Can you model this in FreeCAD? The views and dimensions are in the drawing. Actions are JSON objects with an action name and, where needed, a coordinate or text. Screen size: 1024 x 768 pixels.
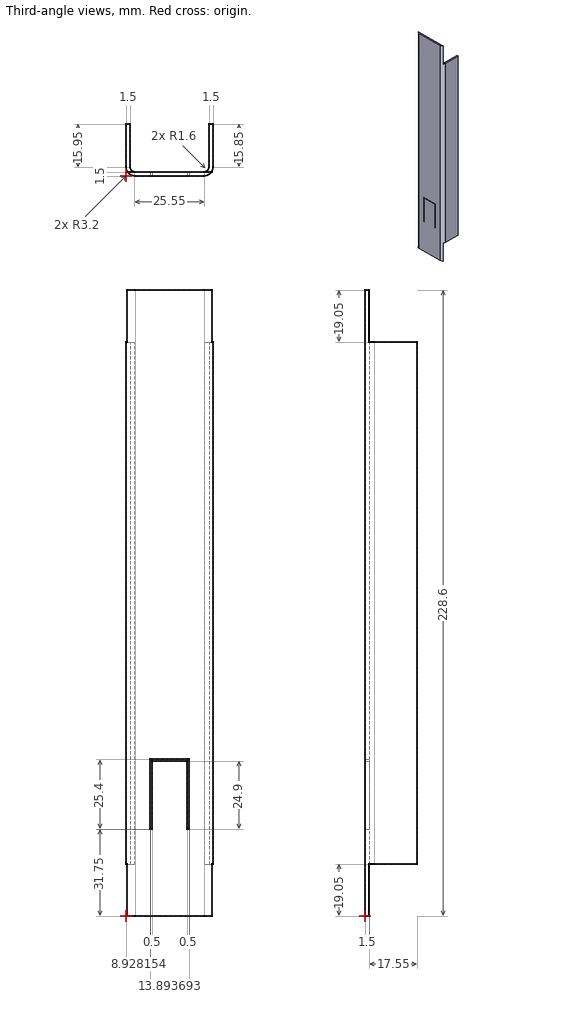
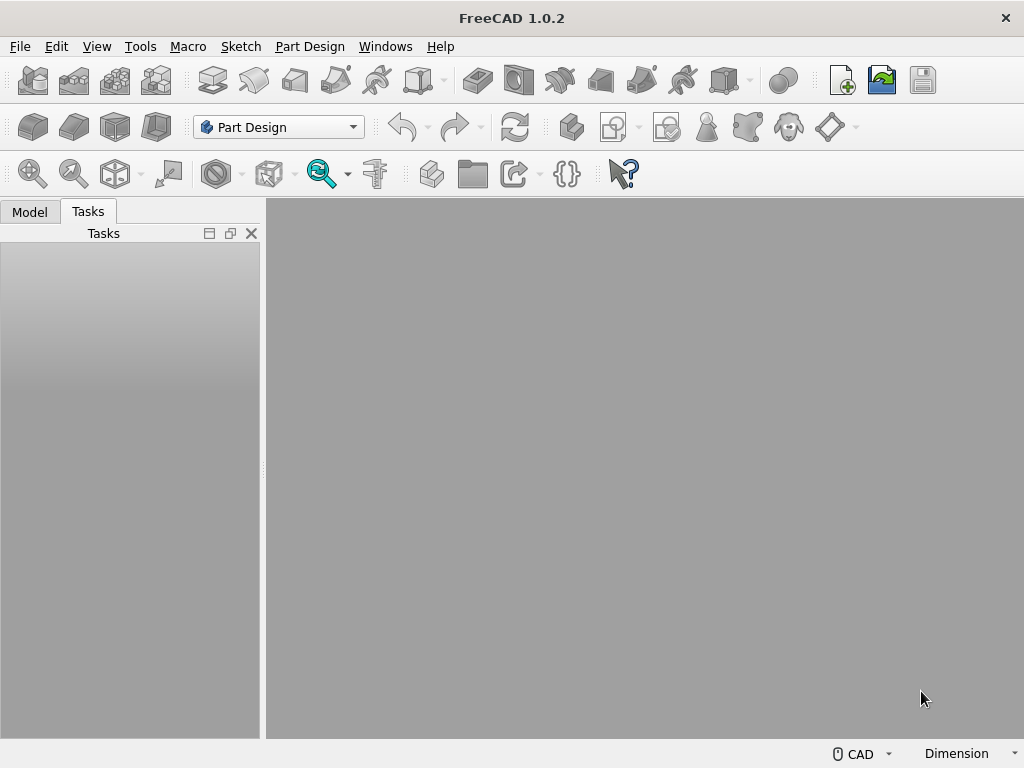
{"action": "left_click", "coordinate": [841, 80]}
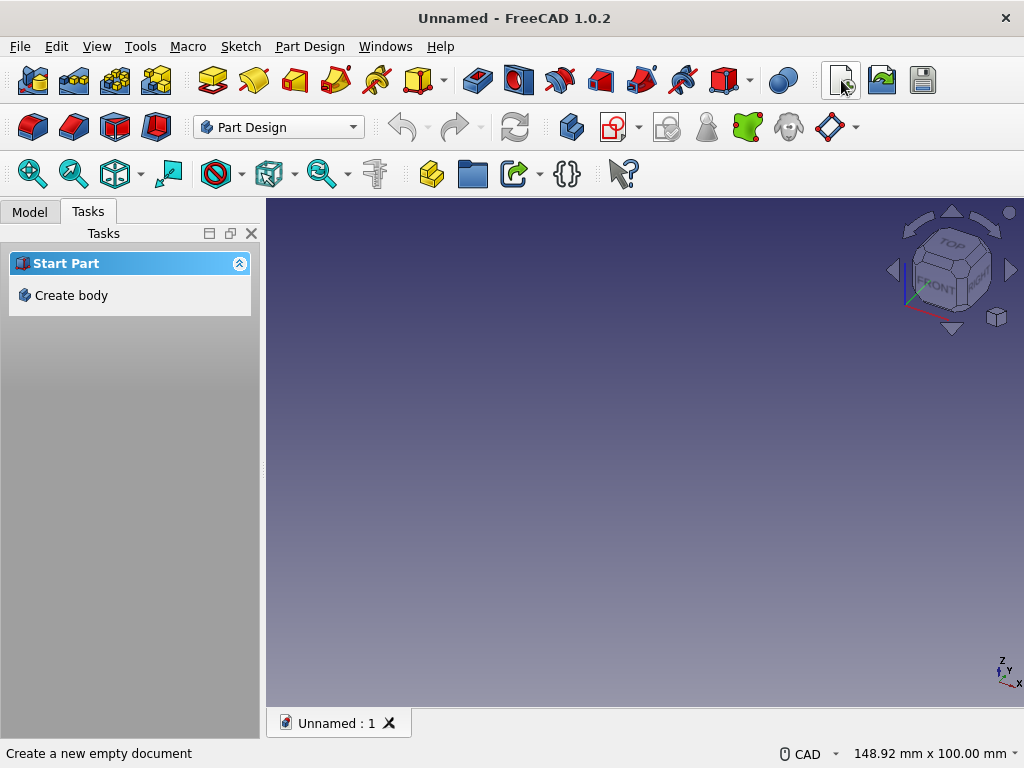
{"action": "left_click", "coordinate": [612, 128]}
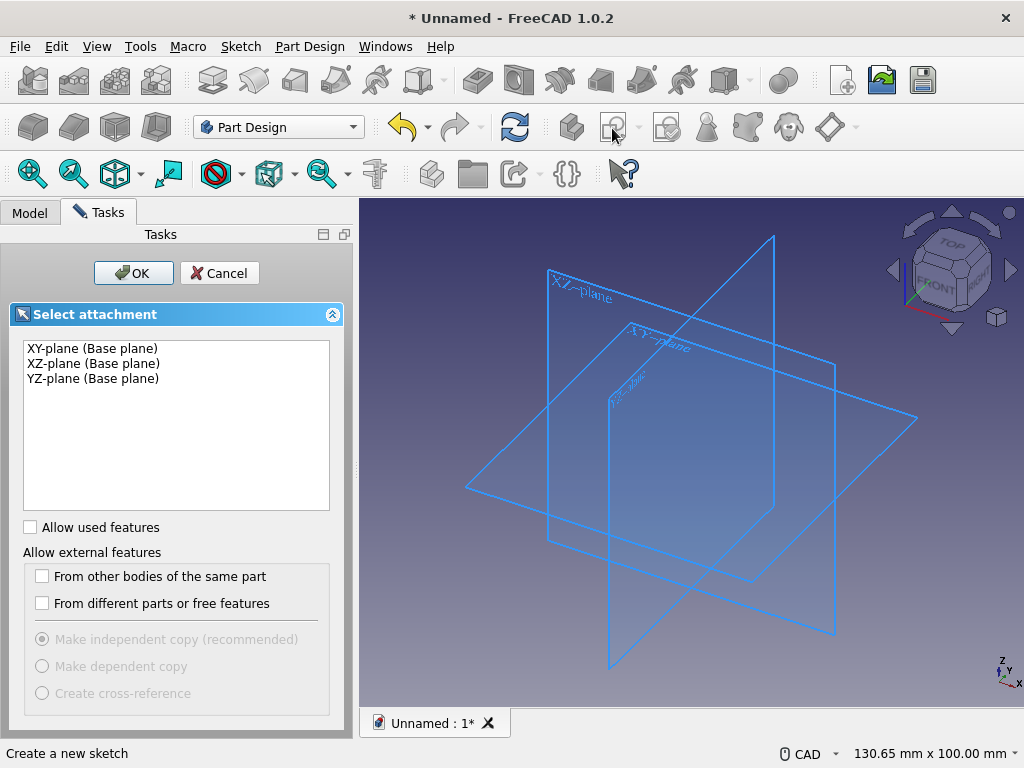
{"action": "left_click", "coordinate": [84, 348]}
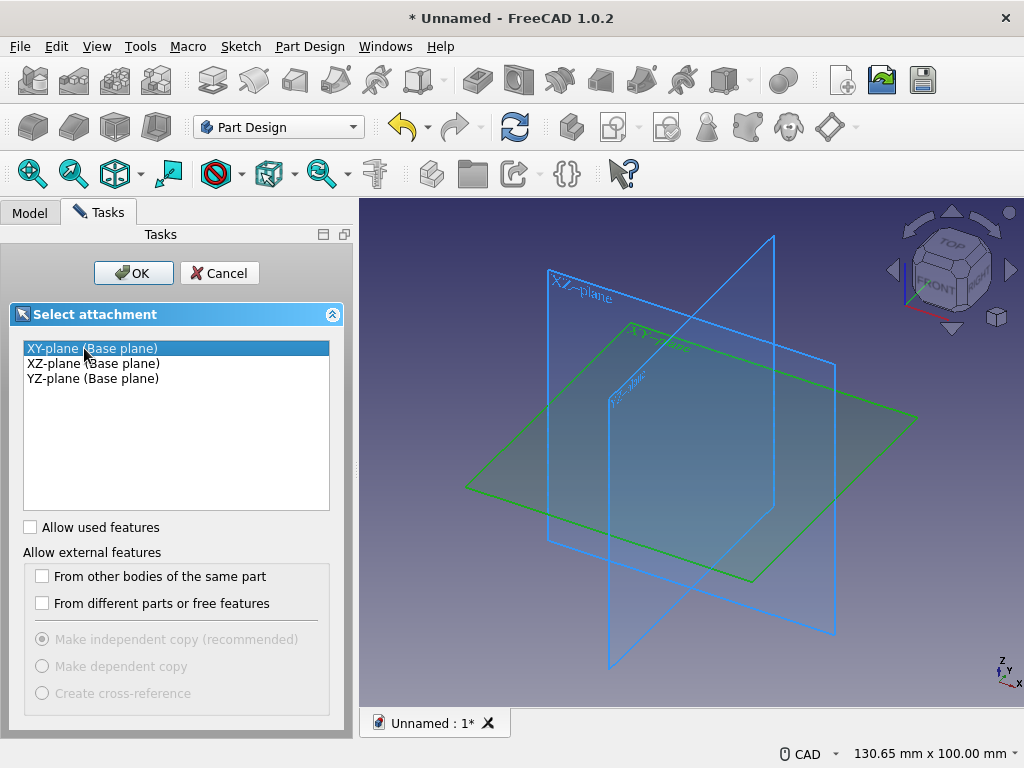
{"action": "left_click", "coordinate": [134, 273]}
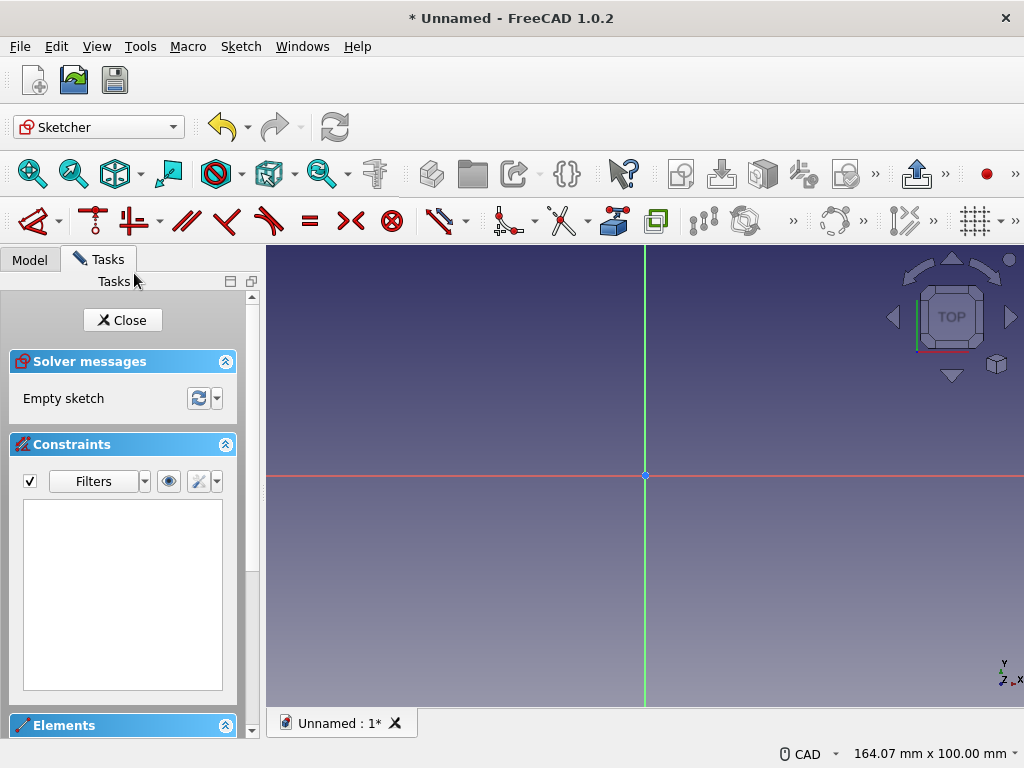
{"action": "scroll", "coordinate": [801, 406], "scroll_direction": "up", "scroll_amount": 5}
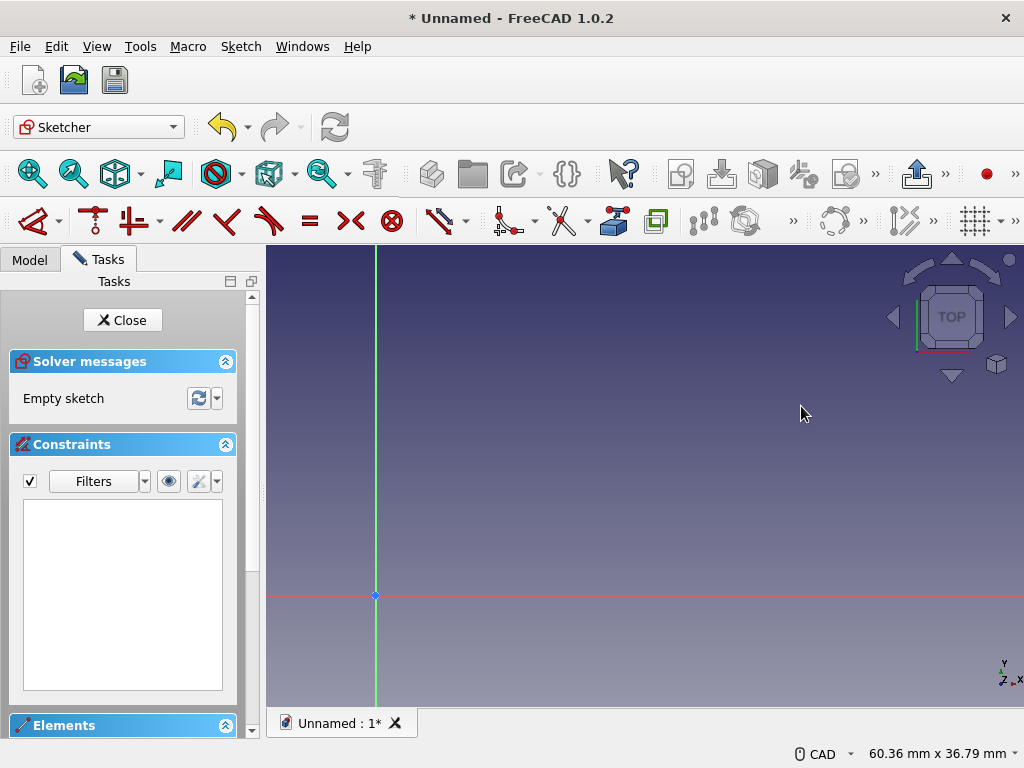
{"action": "key", "text": "g l"}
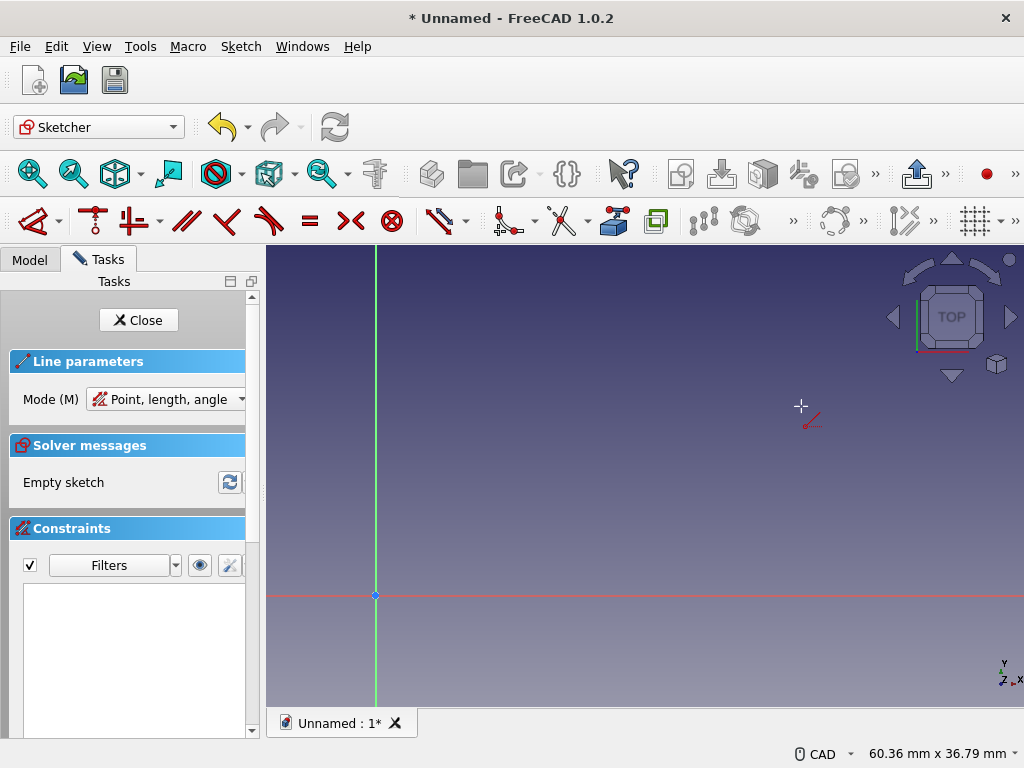
{"action": "left_click", "coordinate": [736, 577]}
{"action": "left_click", "coordinate": [415, 577]}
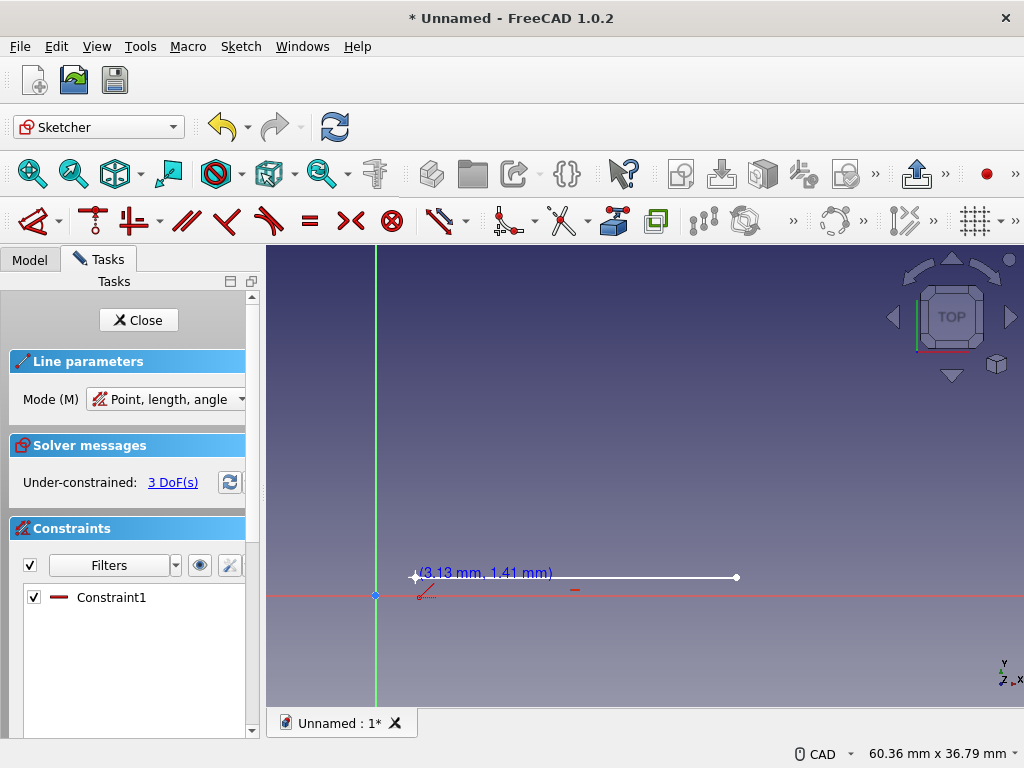
{"action": "key", "text": "g m"}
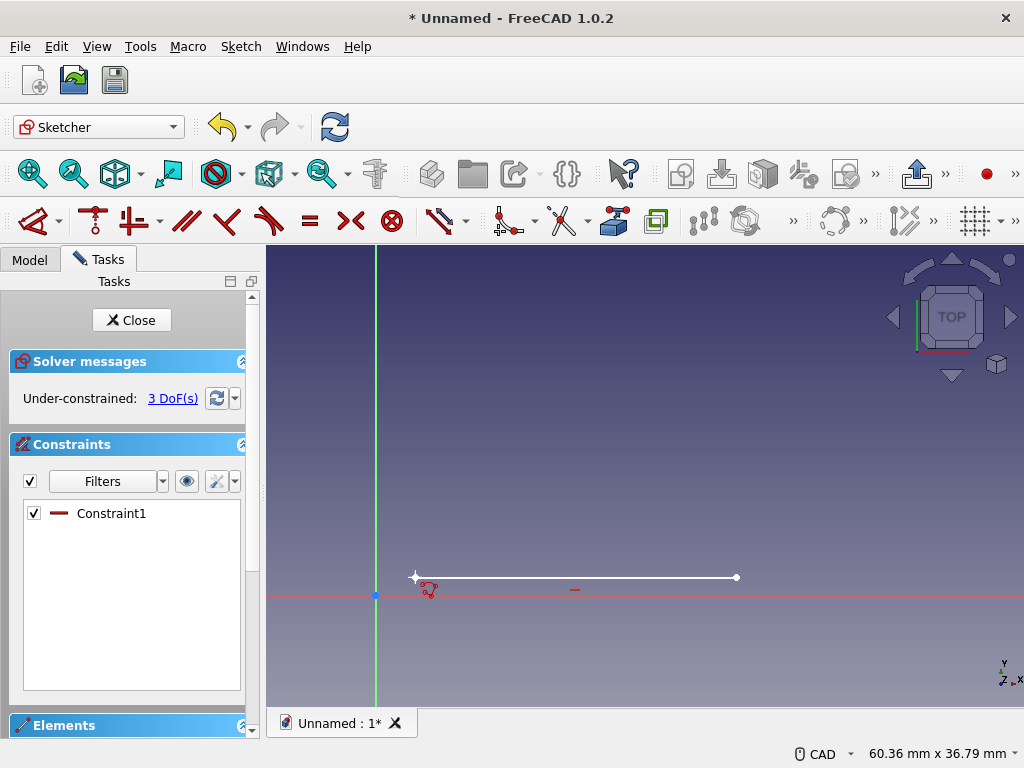
{"action": "left_click", "coordinate": [395, 557]}
{"action": "left_click", "coordinate": [395, 356]}
{"action": "left_click", "coordinate": [376, 356]}
{"action": "left_click", "coordinate": [385, 555]}
{"action": "right_click", "coordinate": [385, 555]}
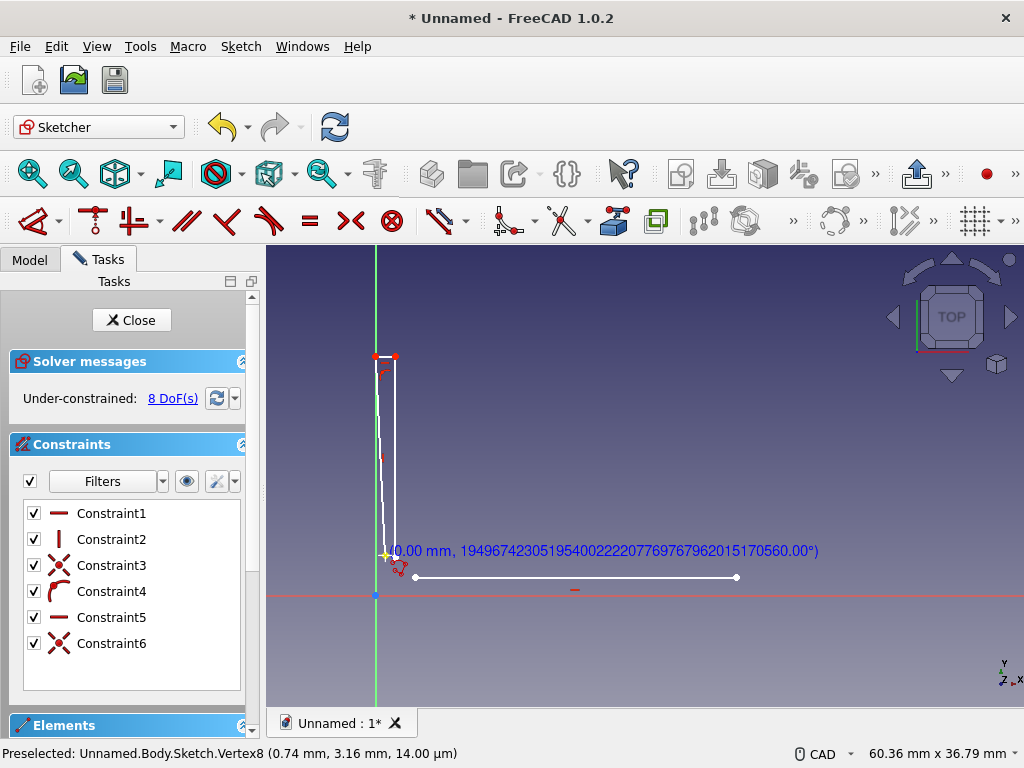
{"action": "key", "text": "g l"}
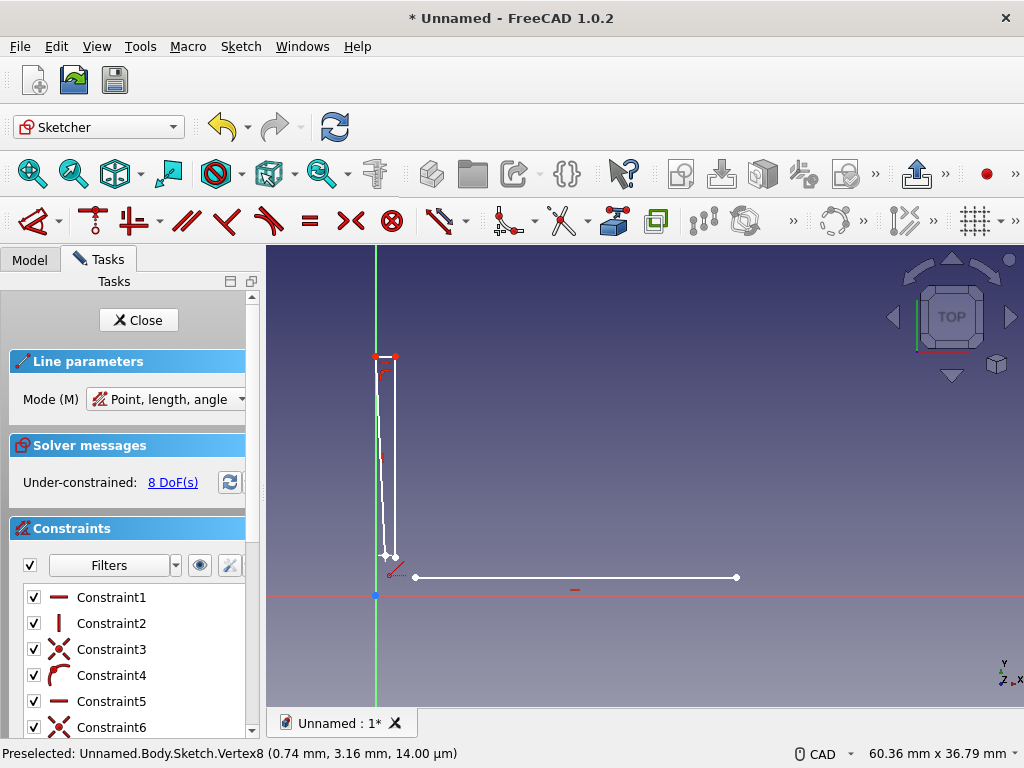
{"action": "left_click", "coordinate": [416, 596]}
{"action": "left_click", "coordinate": [734, 587]}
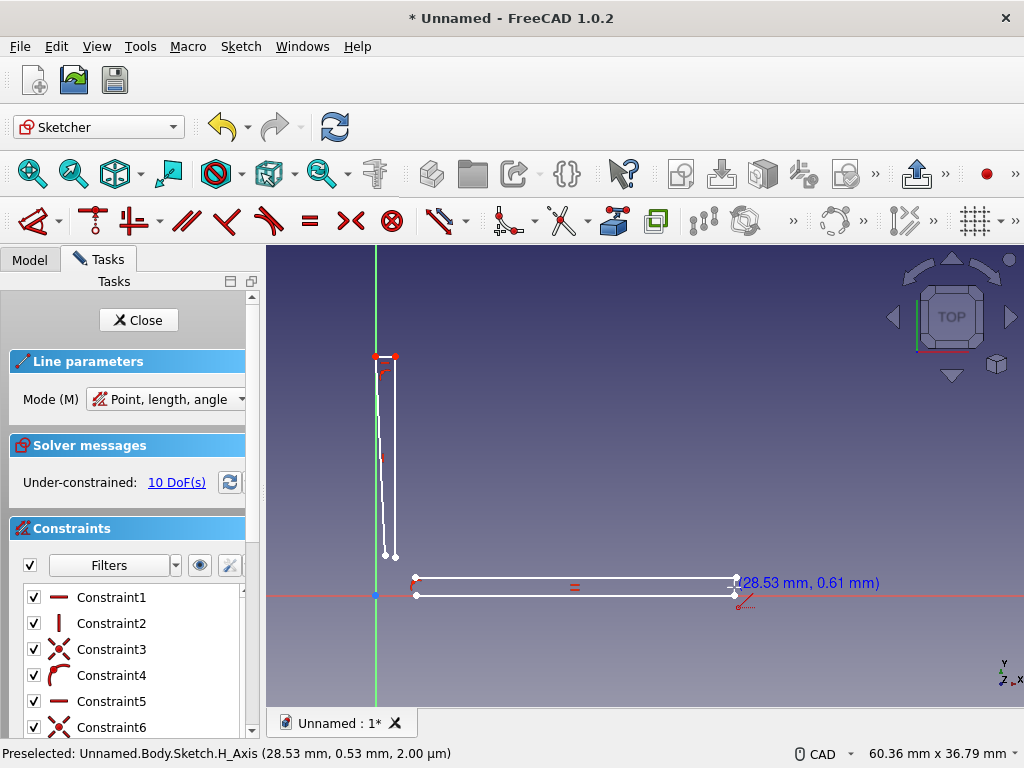
{"action": "key", "text": "g m"}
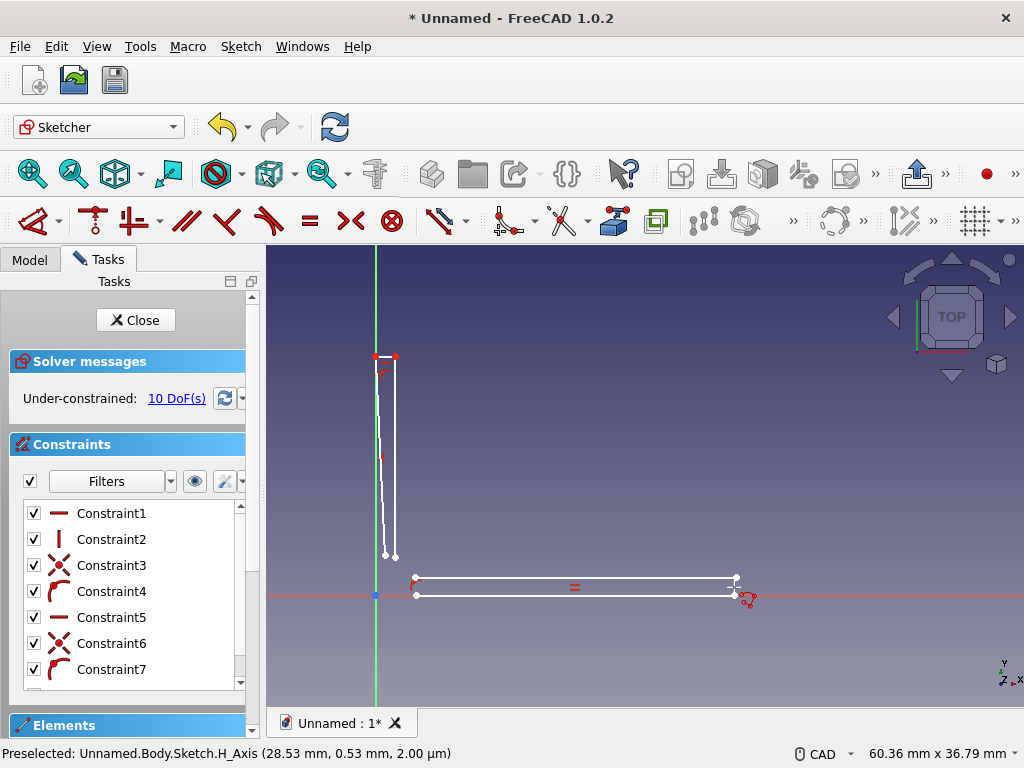
{"action": "left_click", "coordinate": [774, 555]}
{"action": "left_click", "coordinate": [774, 356]}
{"action": "left_click", "coordinate": [756, 356]}
{"action": "left_click", "coordinate": [756, 557]}
{"action": "right_click", "coordinate": [756, 557]}